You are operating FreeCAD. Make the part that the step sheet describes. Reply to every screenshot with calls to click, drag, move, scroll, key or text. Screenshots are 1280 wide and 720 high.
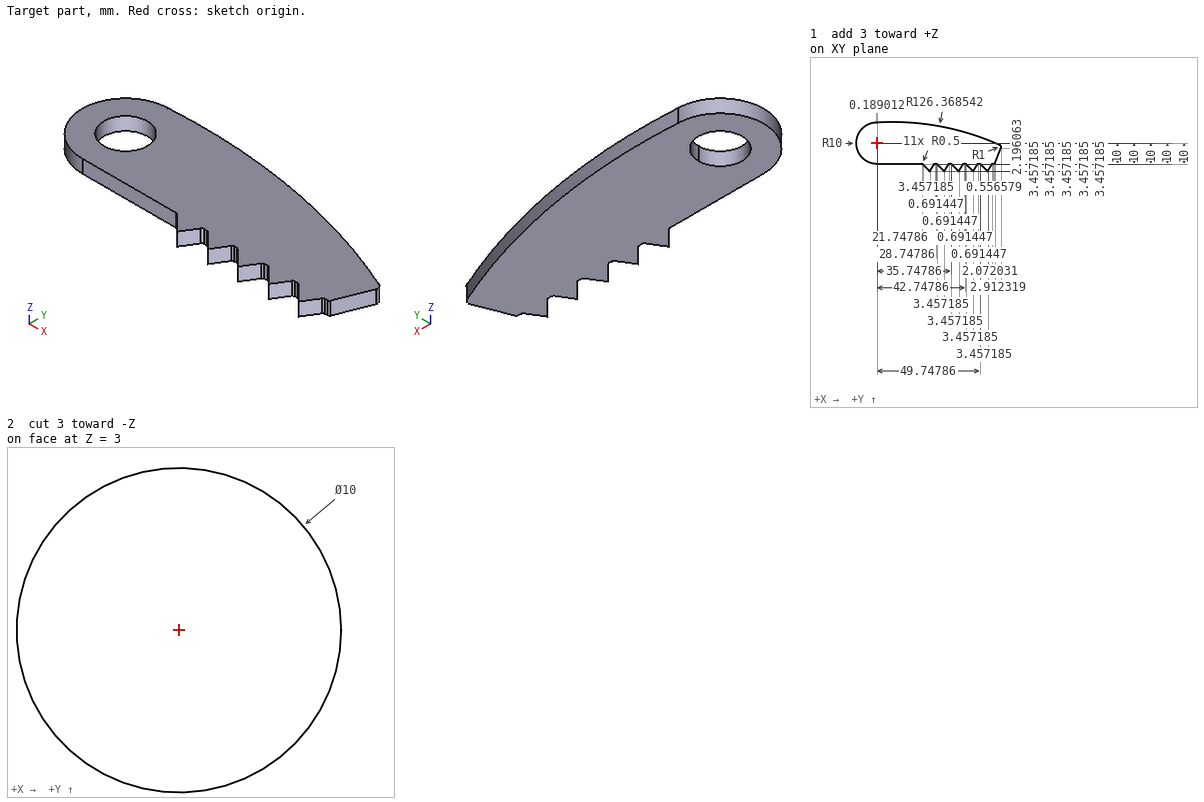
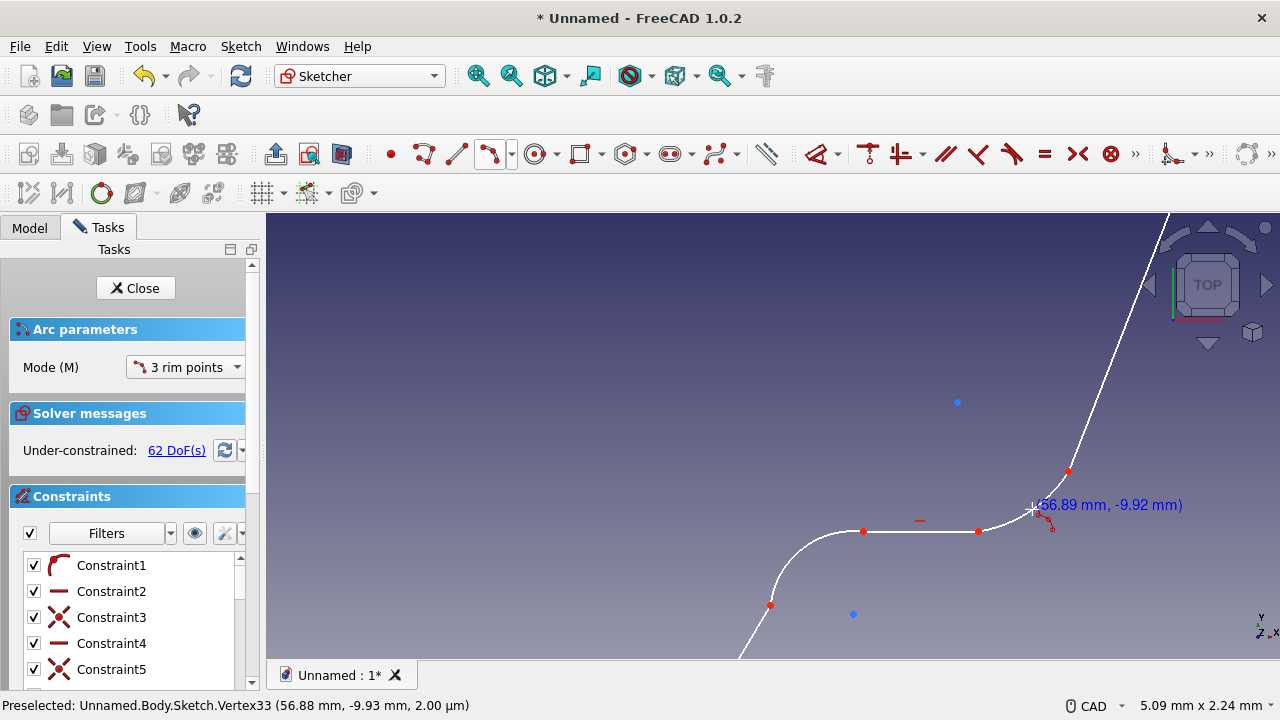
scroll(1021, 517, down, 15)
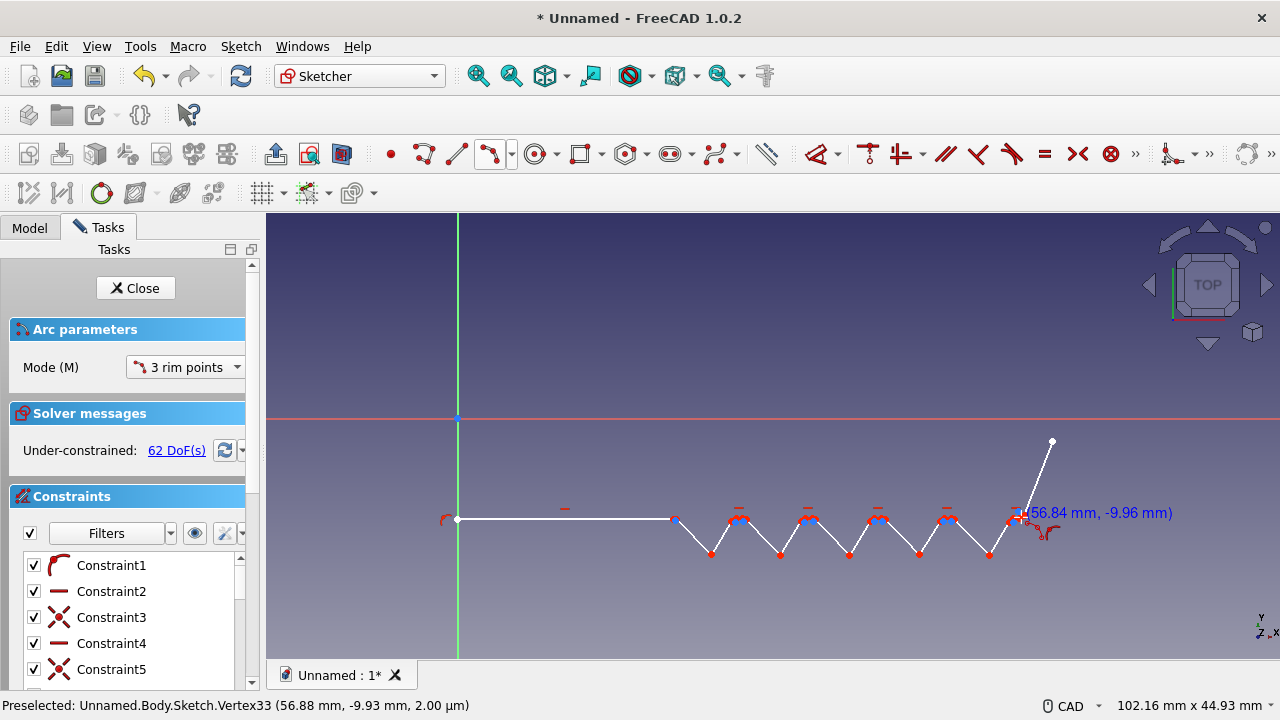
click(1053, 441)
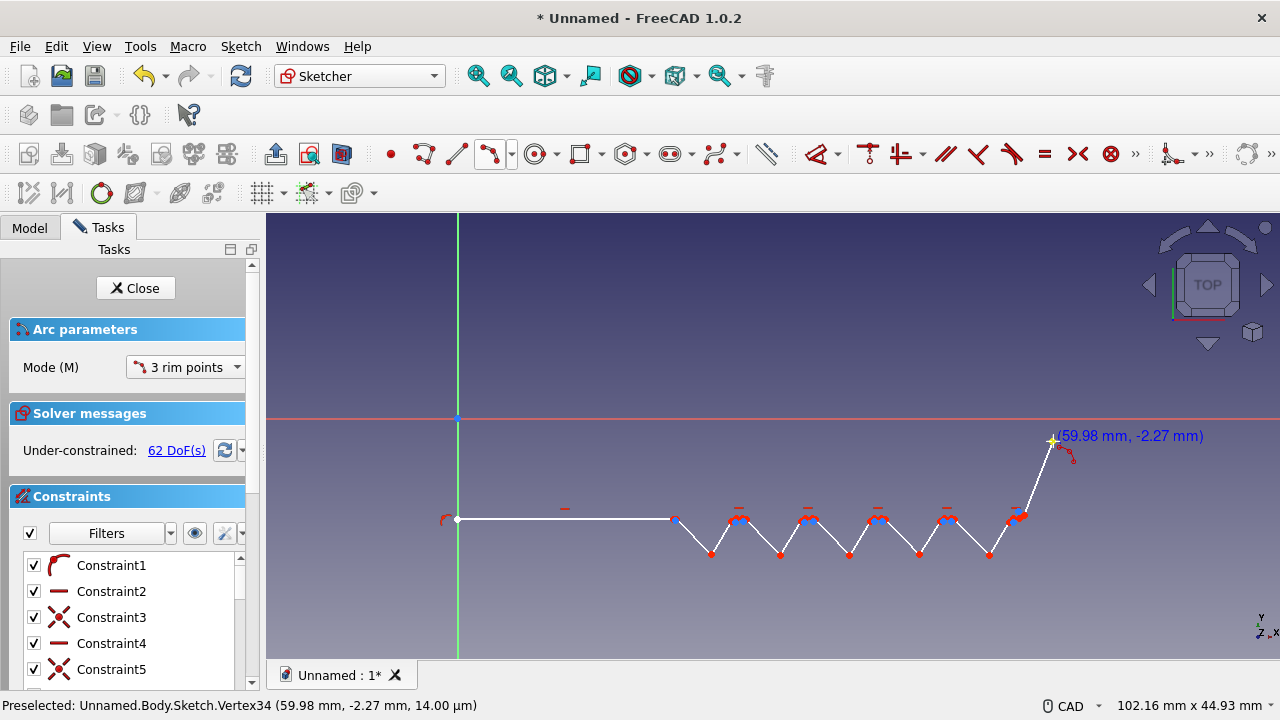
scroll(1048, 428, up, 3)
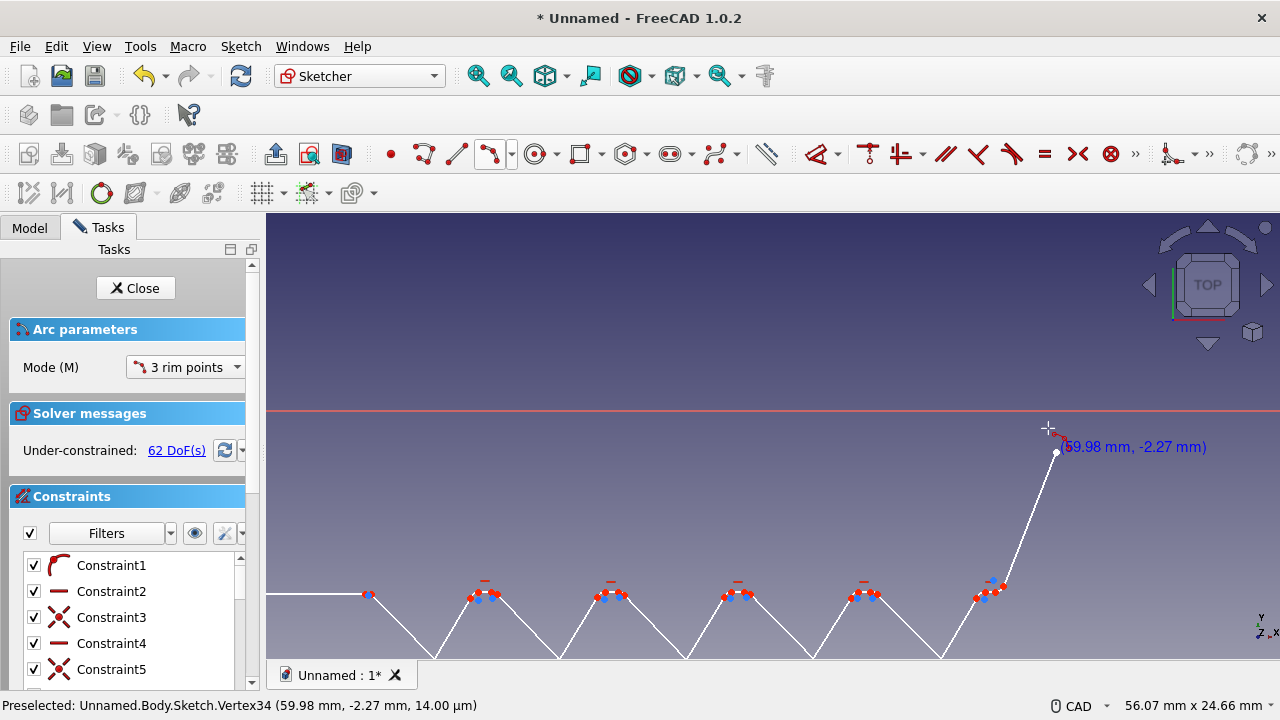
click(1047, 428)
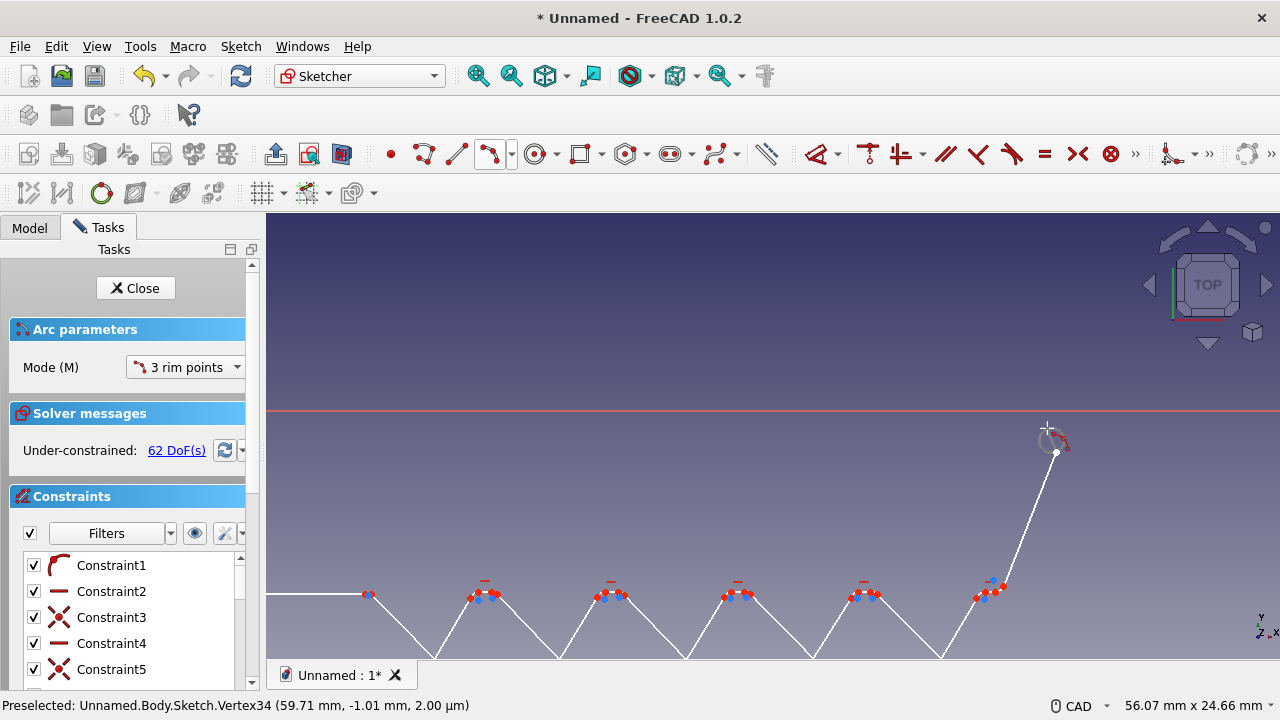
scroll(1056, 437, up, 6)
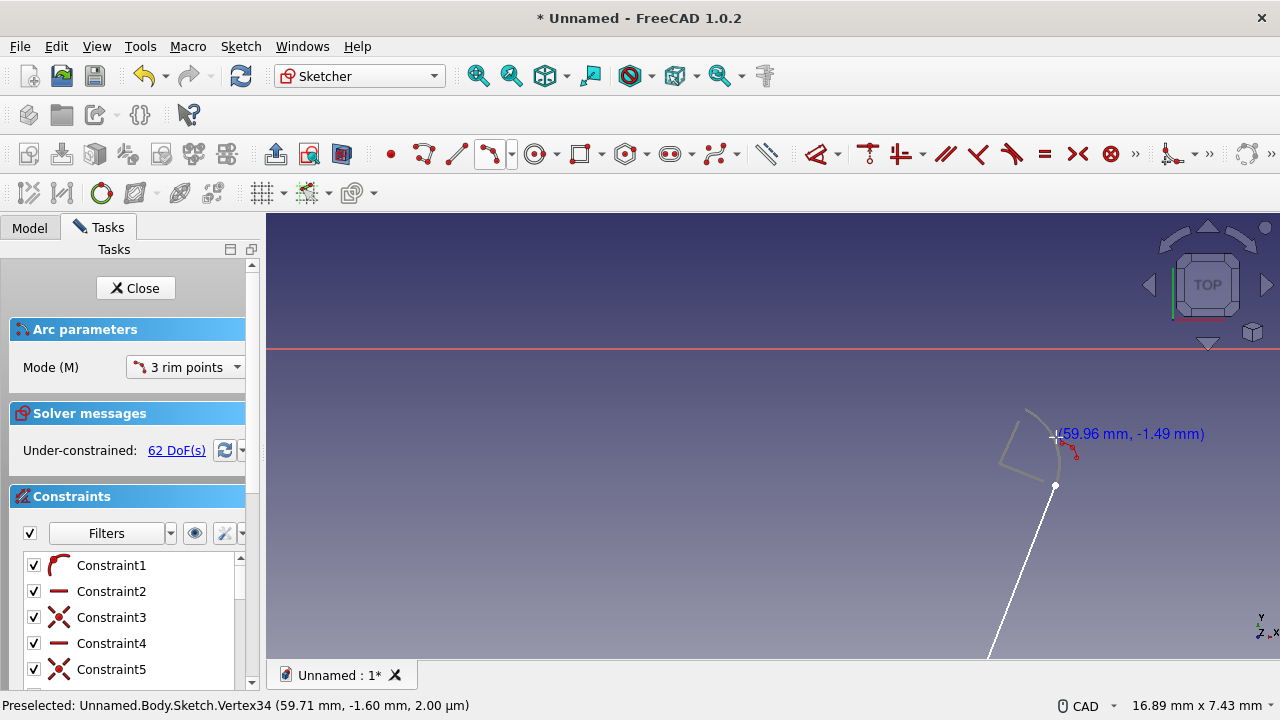
click(1055, 437)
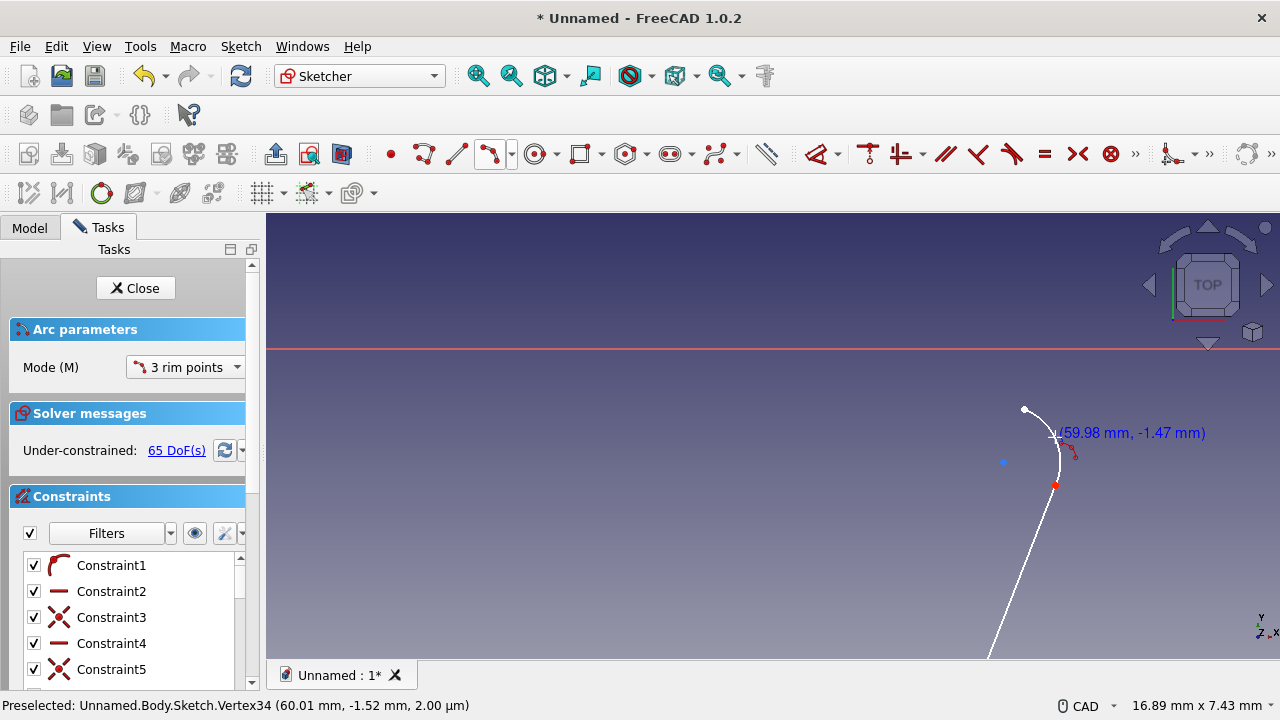
scroll(978, 433, down, 10)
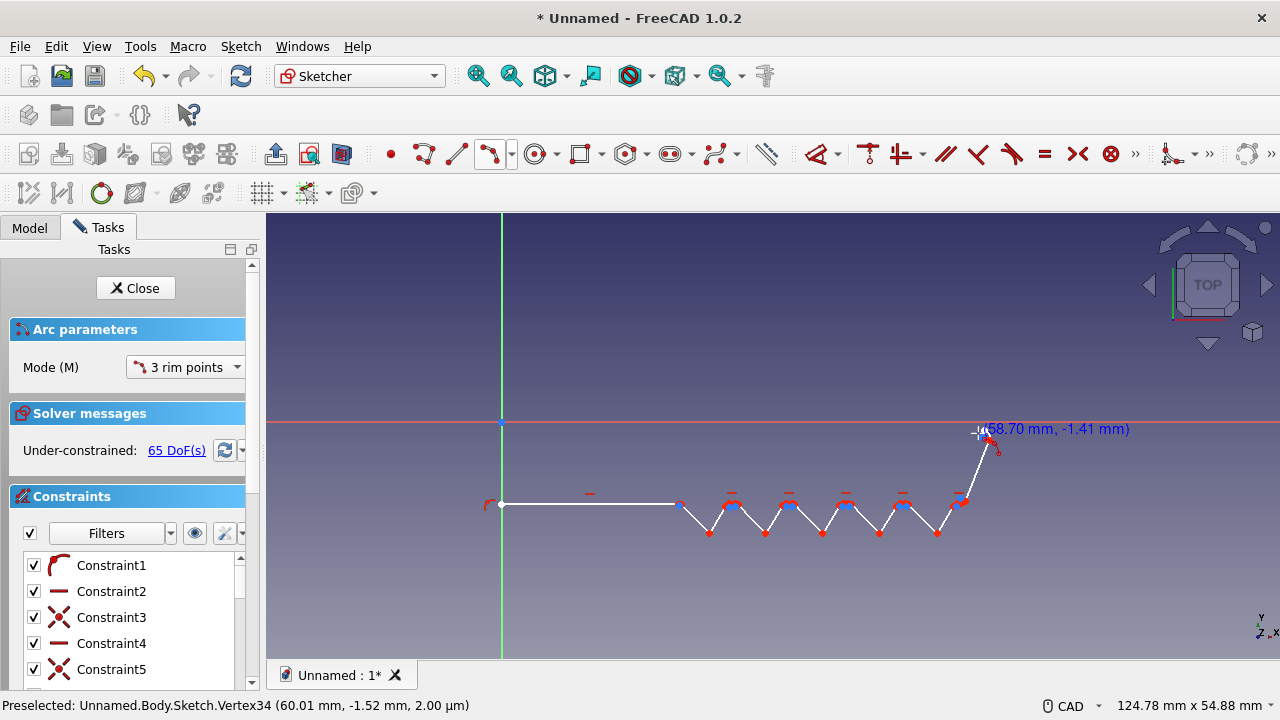
scroll(985, 430, up, 4)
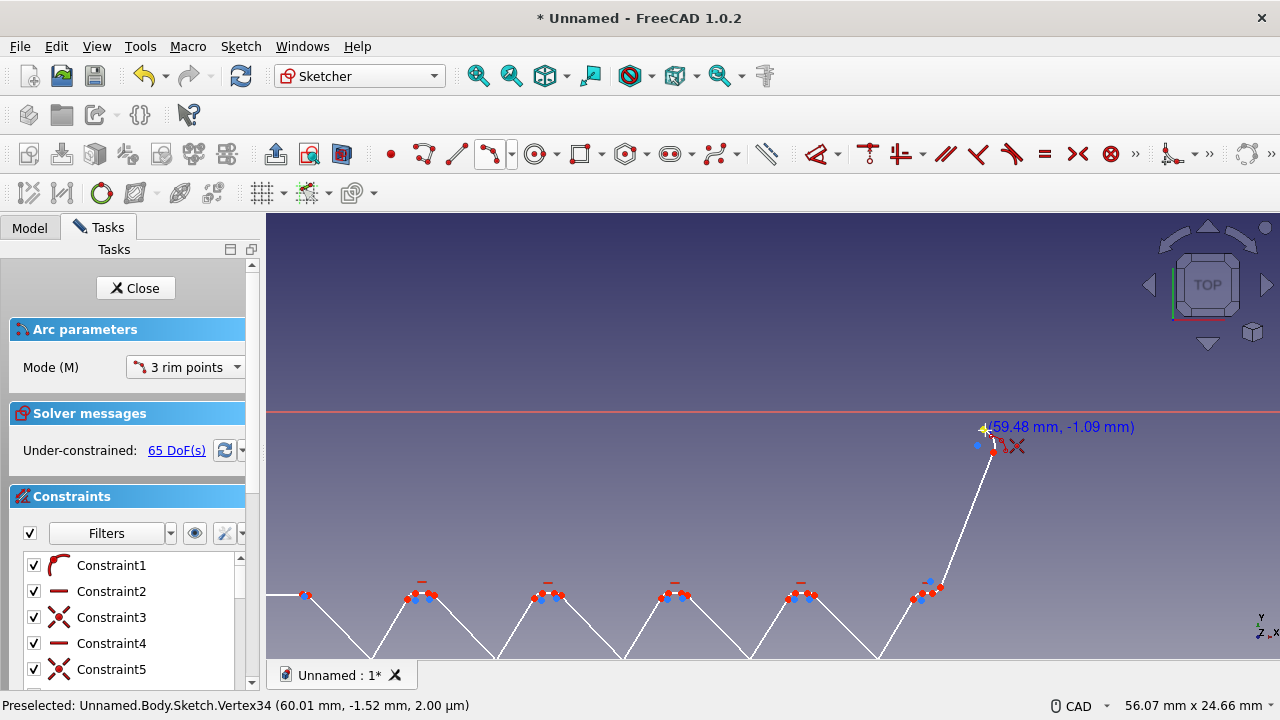
click(984, 430)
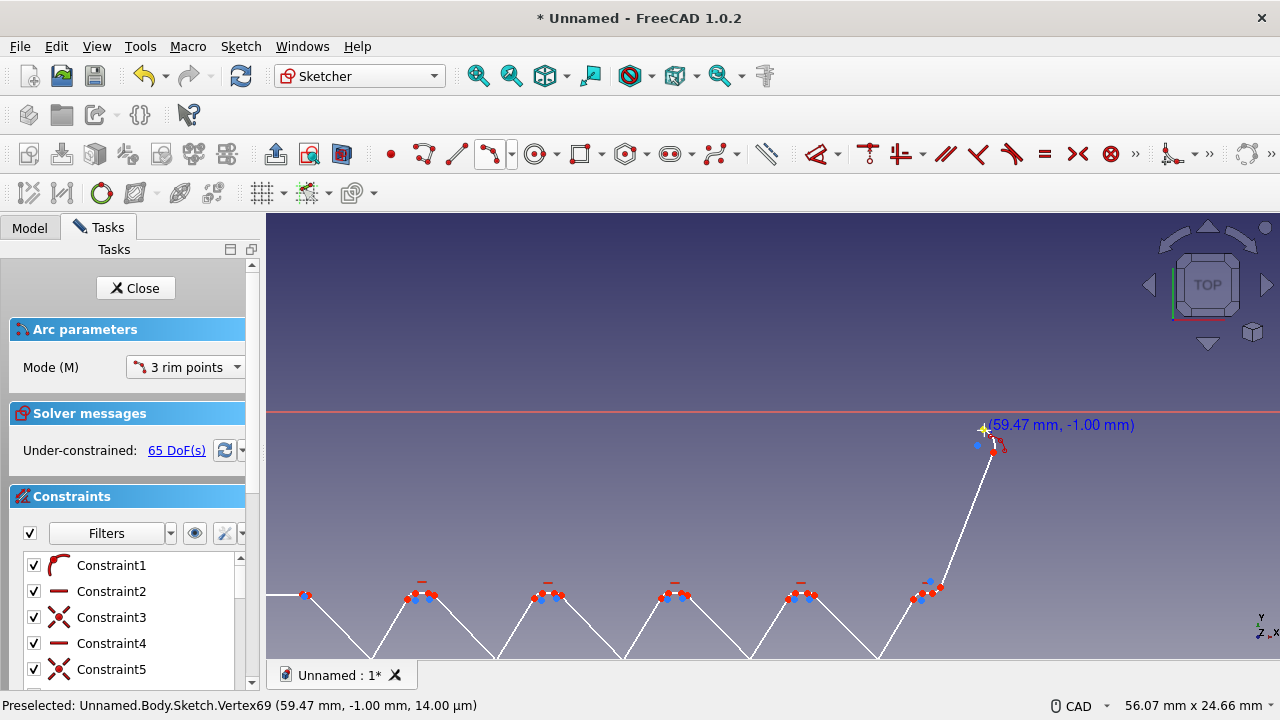
scroll(985, 429, down, 4)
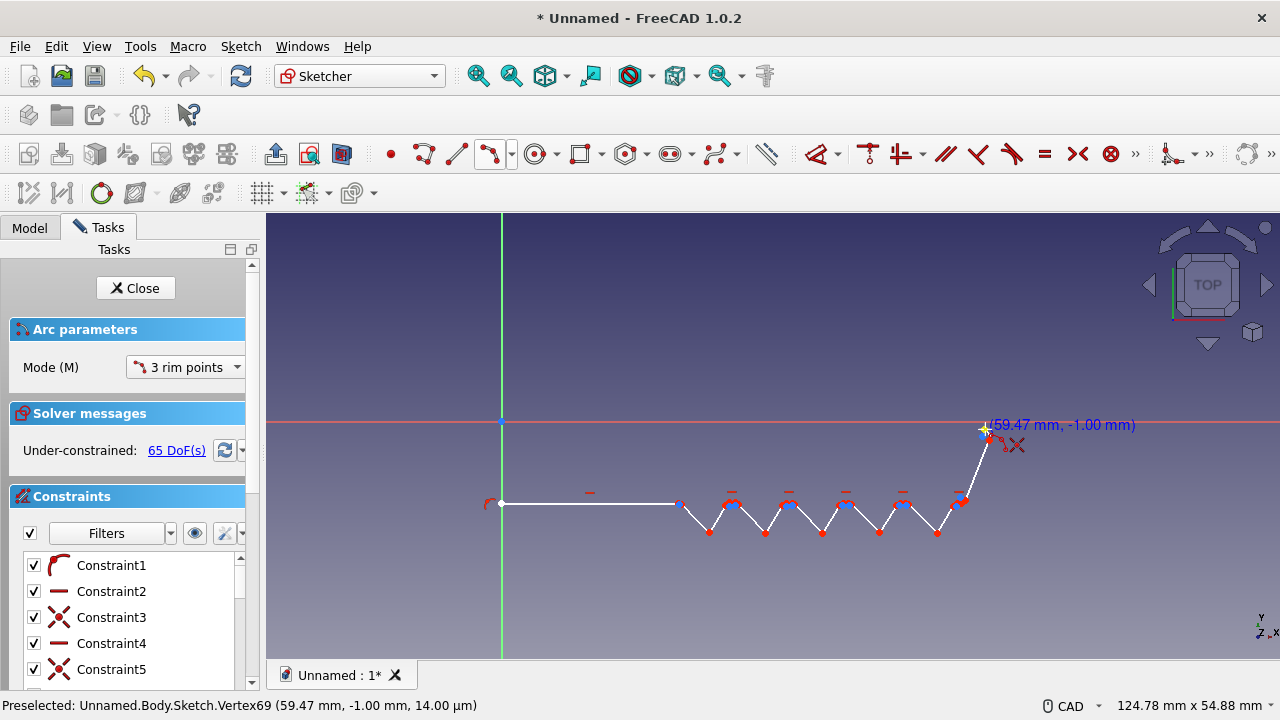
scroll(500, 340, up, 12)